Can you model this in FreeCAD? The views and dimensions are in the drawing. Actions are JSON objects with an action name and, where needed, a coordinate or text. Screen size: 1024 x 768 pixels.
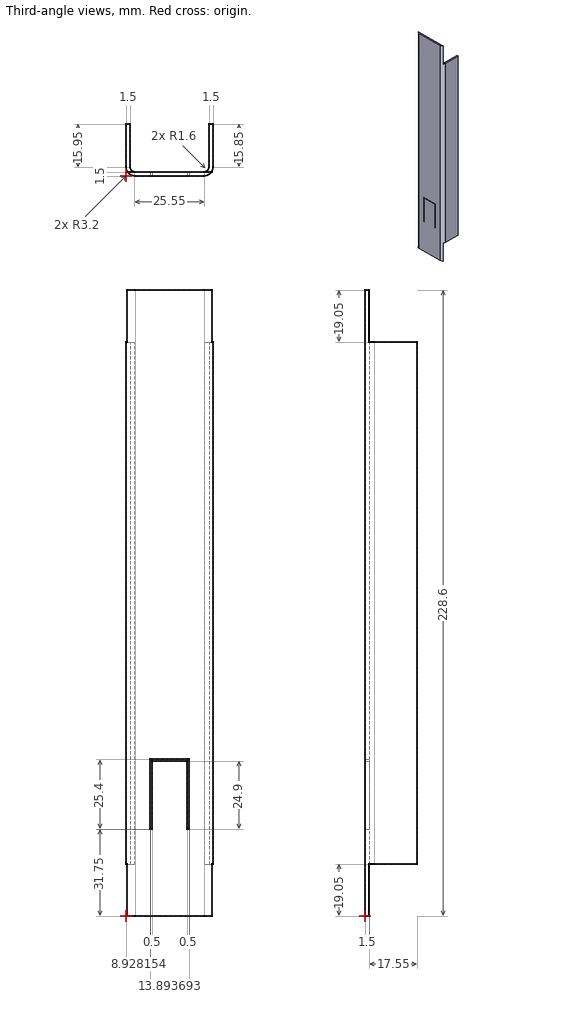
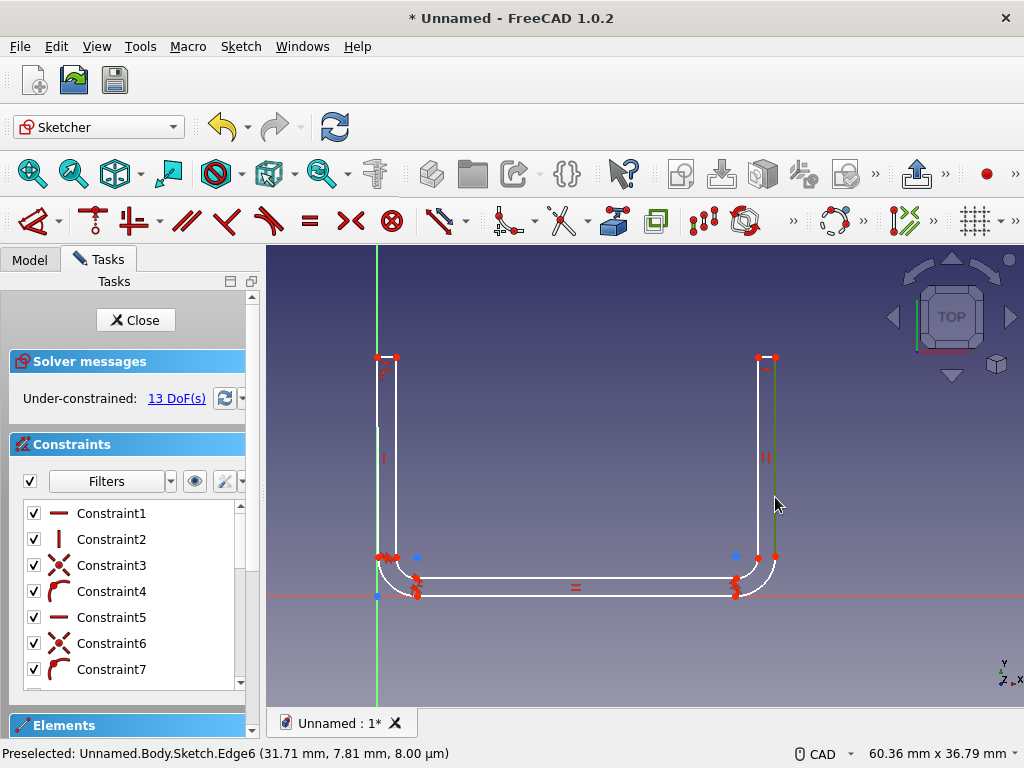
{"action": "left_click", "coordinate": [771, 574]}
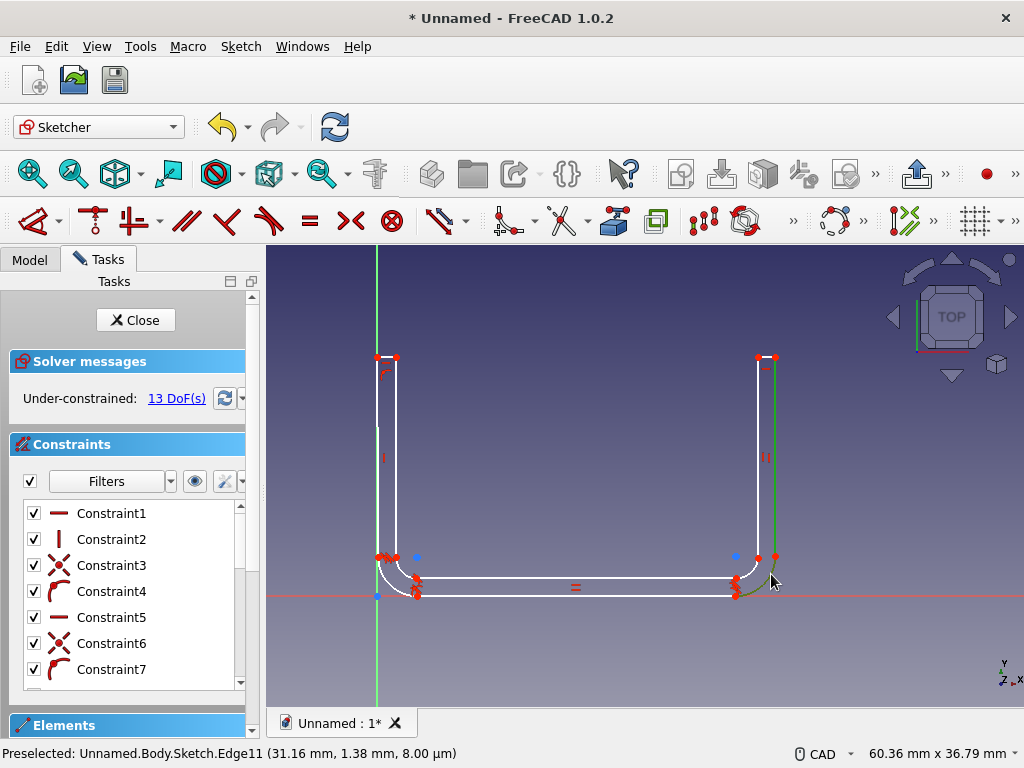
{"action": "left_click", "coordinate": [269, 222]}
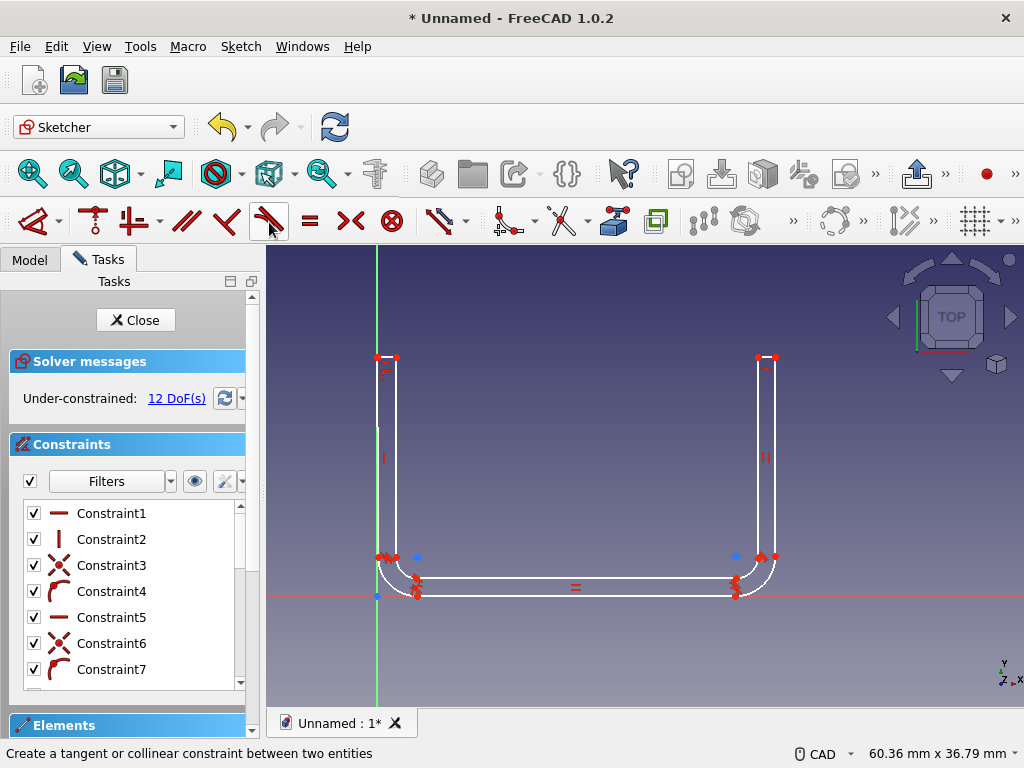
{"action": "left_click", "coordinate": [758, 418]}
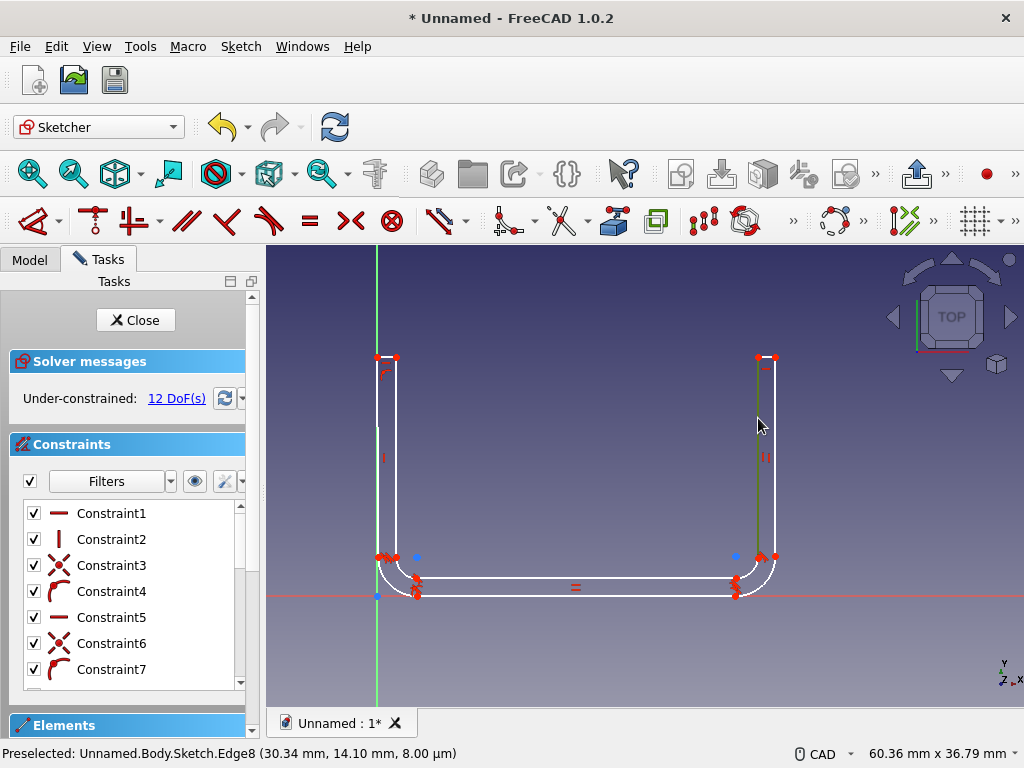
{"action": "scroll", "coordinate": [745, 576], "scroll_direction": "up", "scroll_amount": 2}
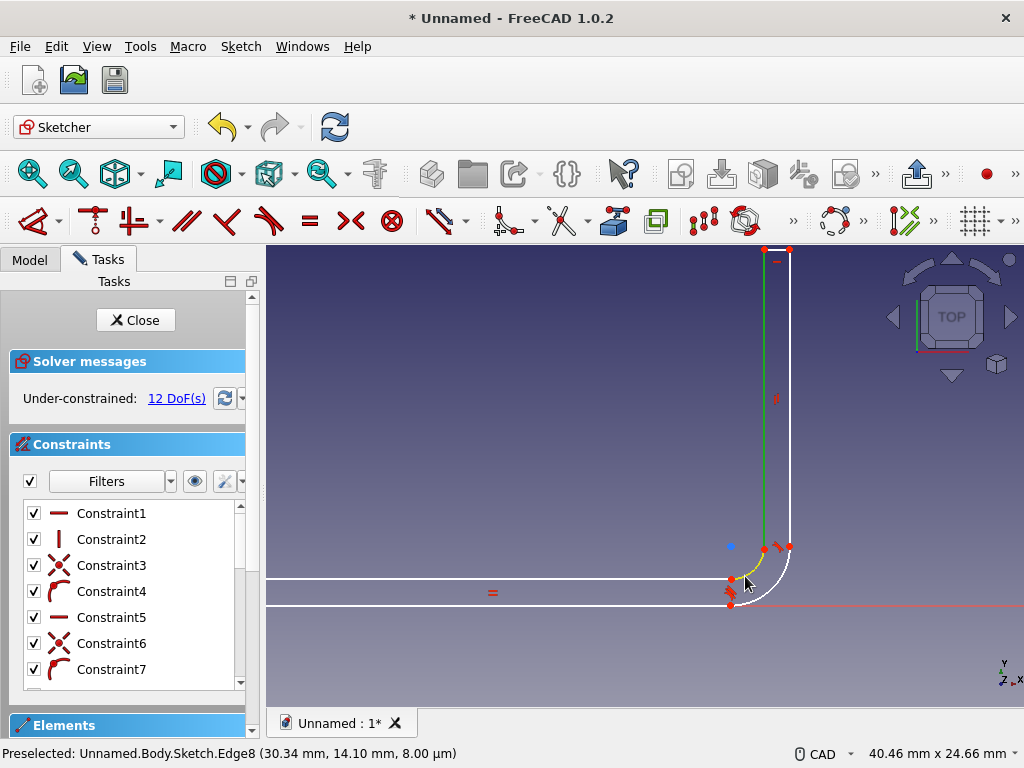
{"action": "left_click", "coordinate": [745, 576]}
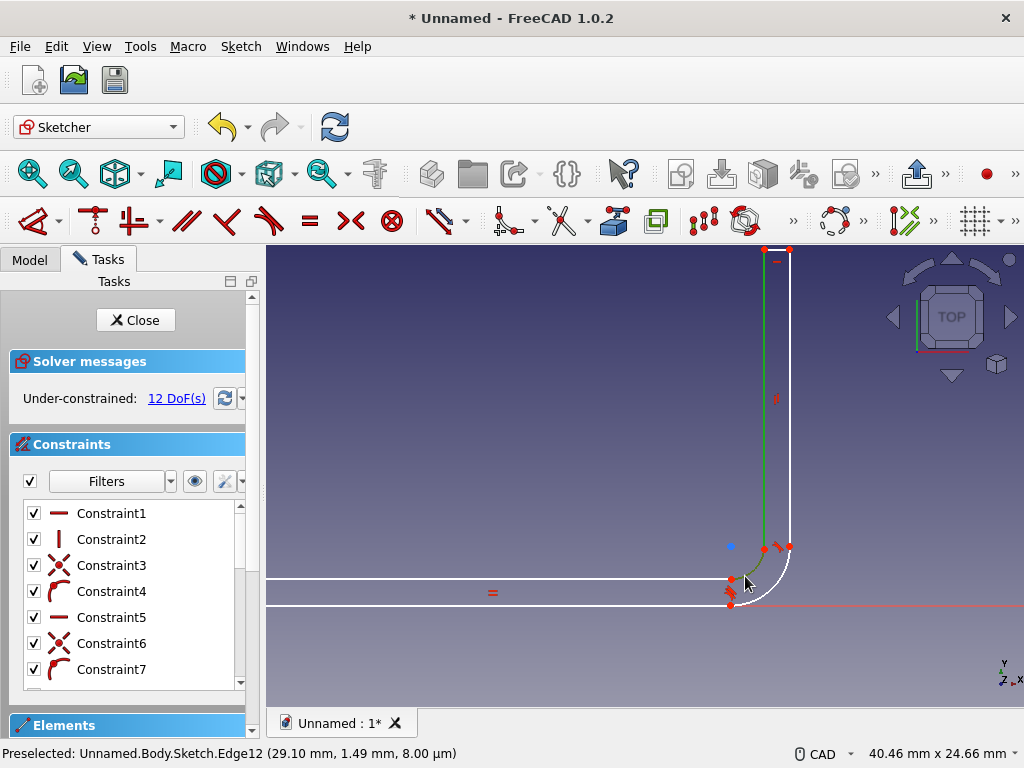
{"action": "left_click", "coordinate": [269, 222]}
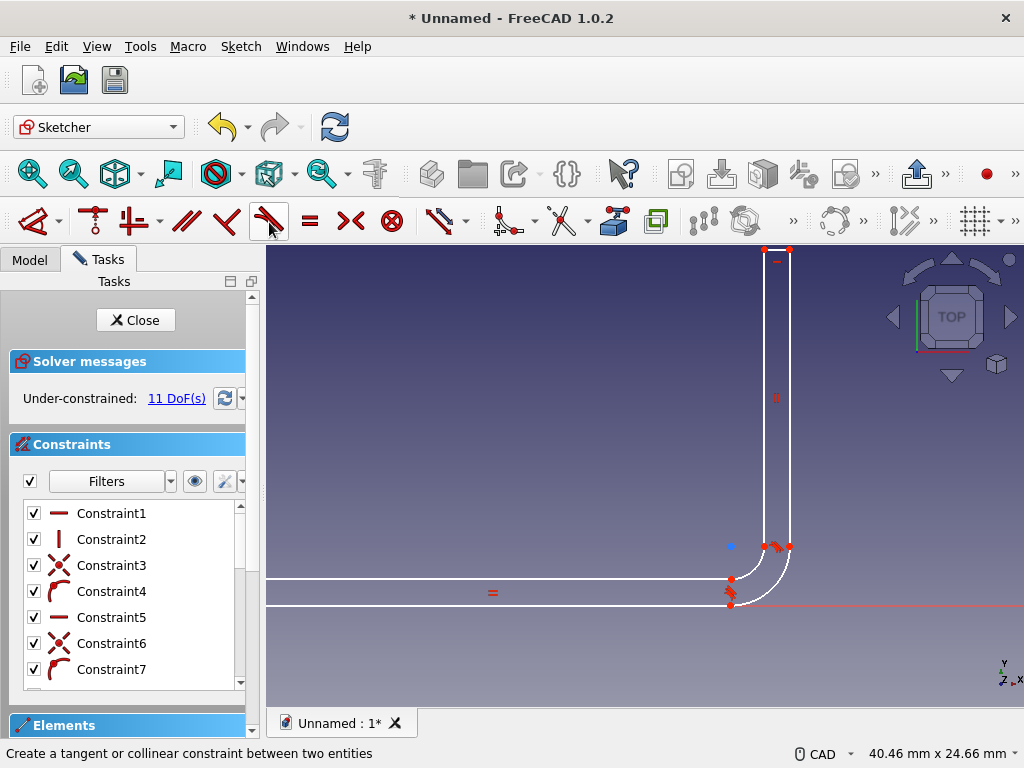
{"action": "scroll", "coordinate": [746, 575], "scroll_direction": "down", "scroll_amount": 2}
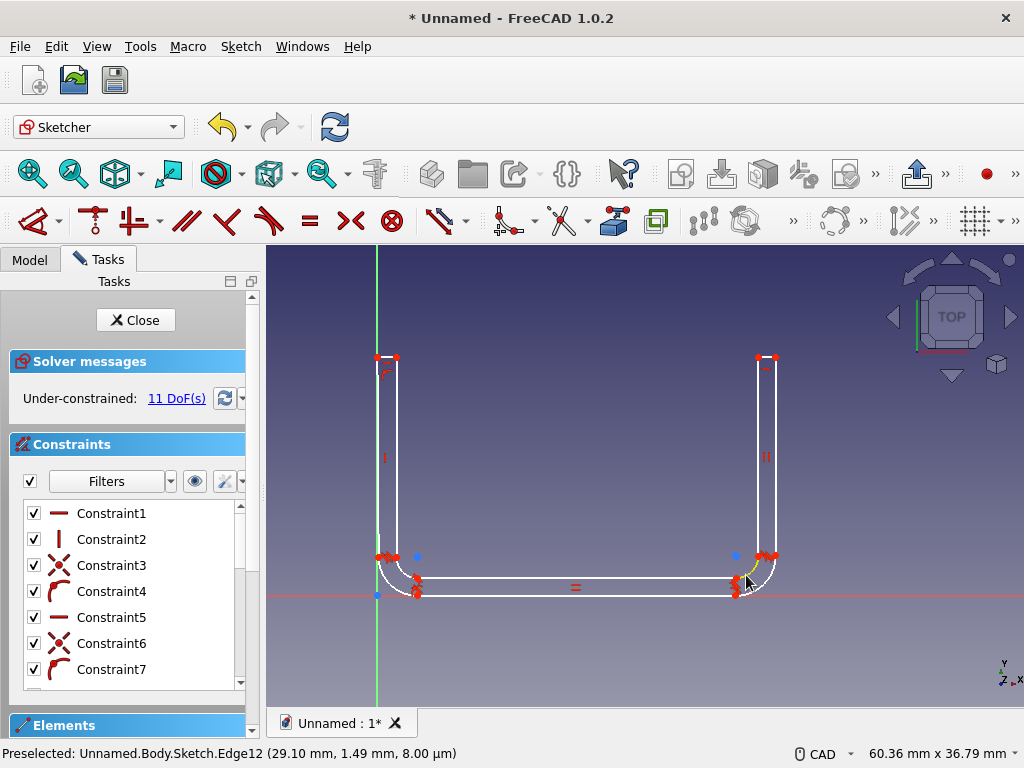
{"action": "left_click", "coordinate": [378, 417]}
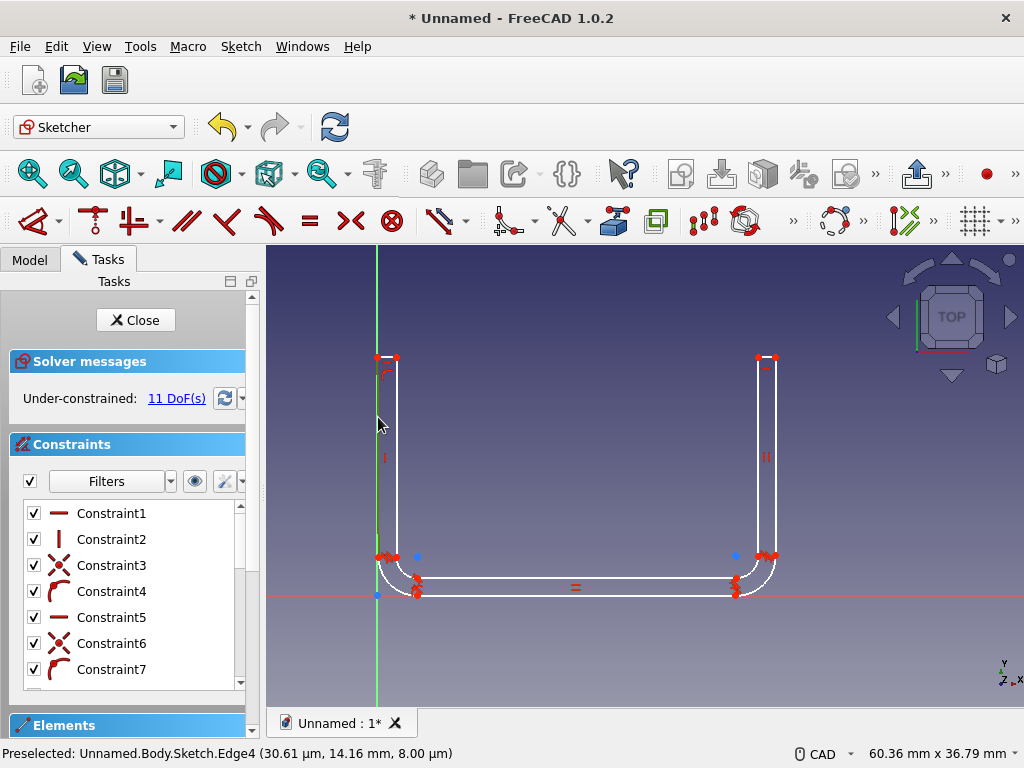
{"action": "left_click", "coordinate": [160, 222]}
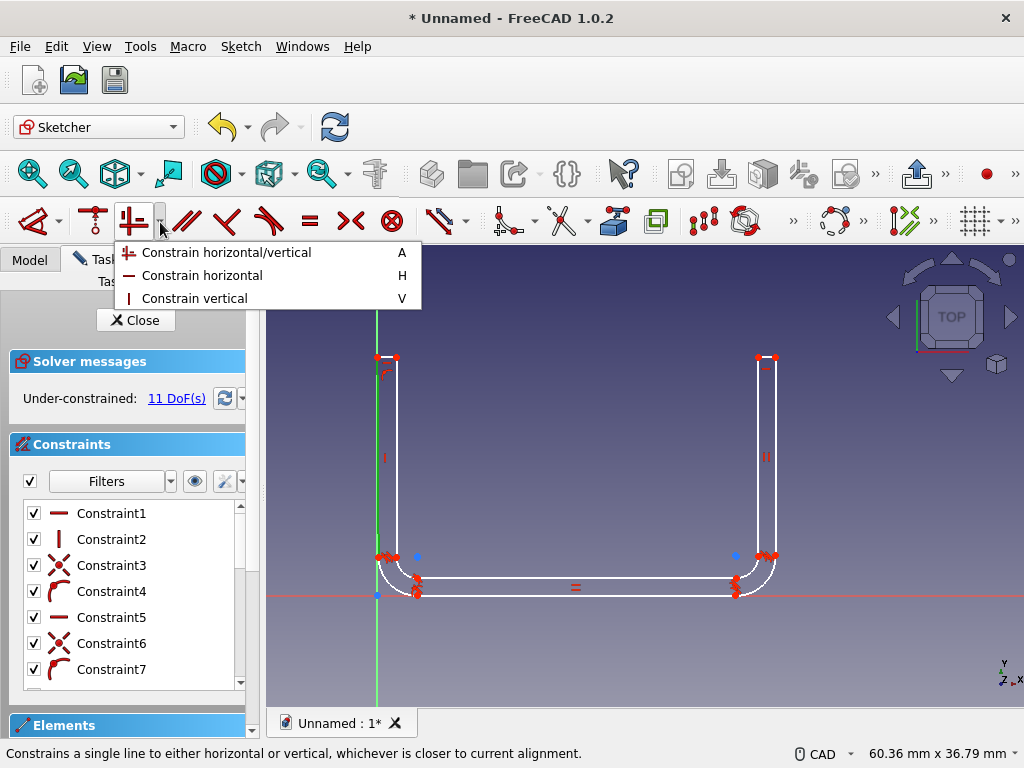
{"action": "left_click", "coordinate": [268, 298]}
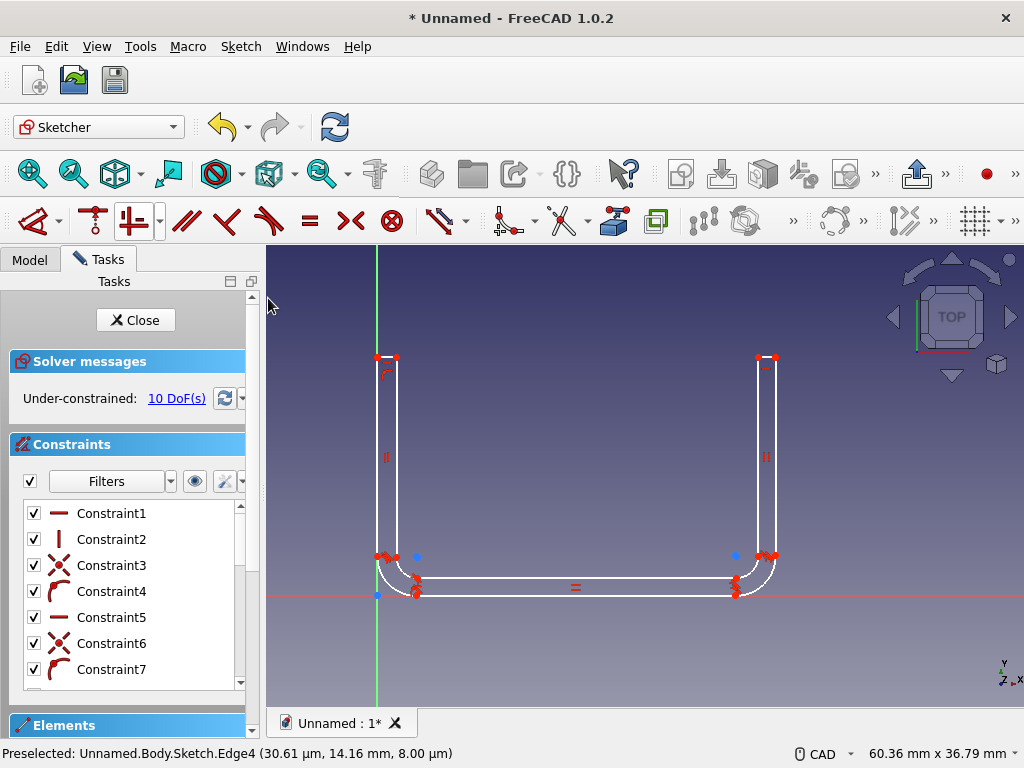
{"action": "left_click", "coordinate": [389, 584]}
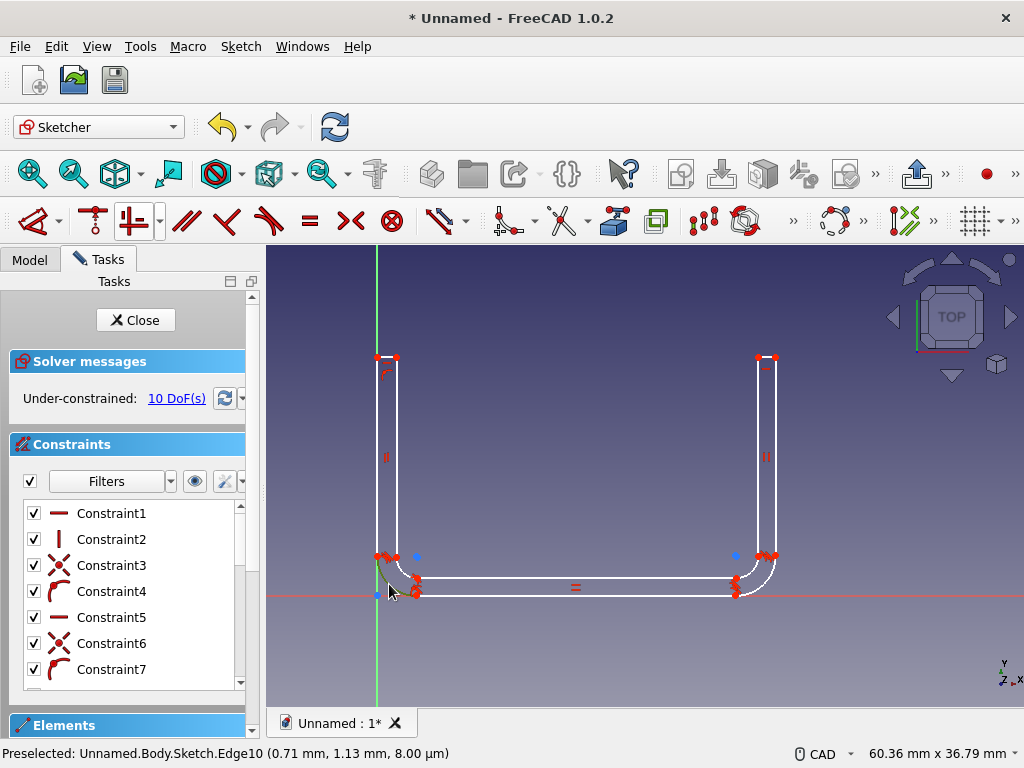
{"action": "left_click", "coordinate": [771, 574]}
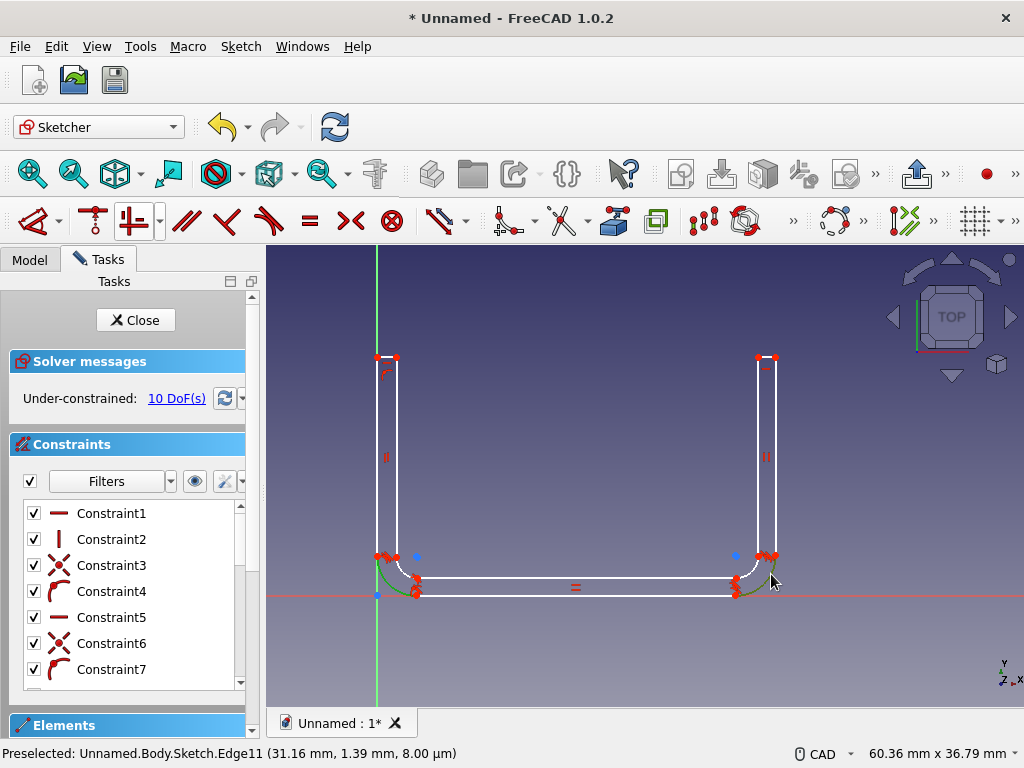
{"action": "left_click", "coordinate": [310, 222]}